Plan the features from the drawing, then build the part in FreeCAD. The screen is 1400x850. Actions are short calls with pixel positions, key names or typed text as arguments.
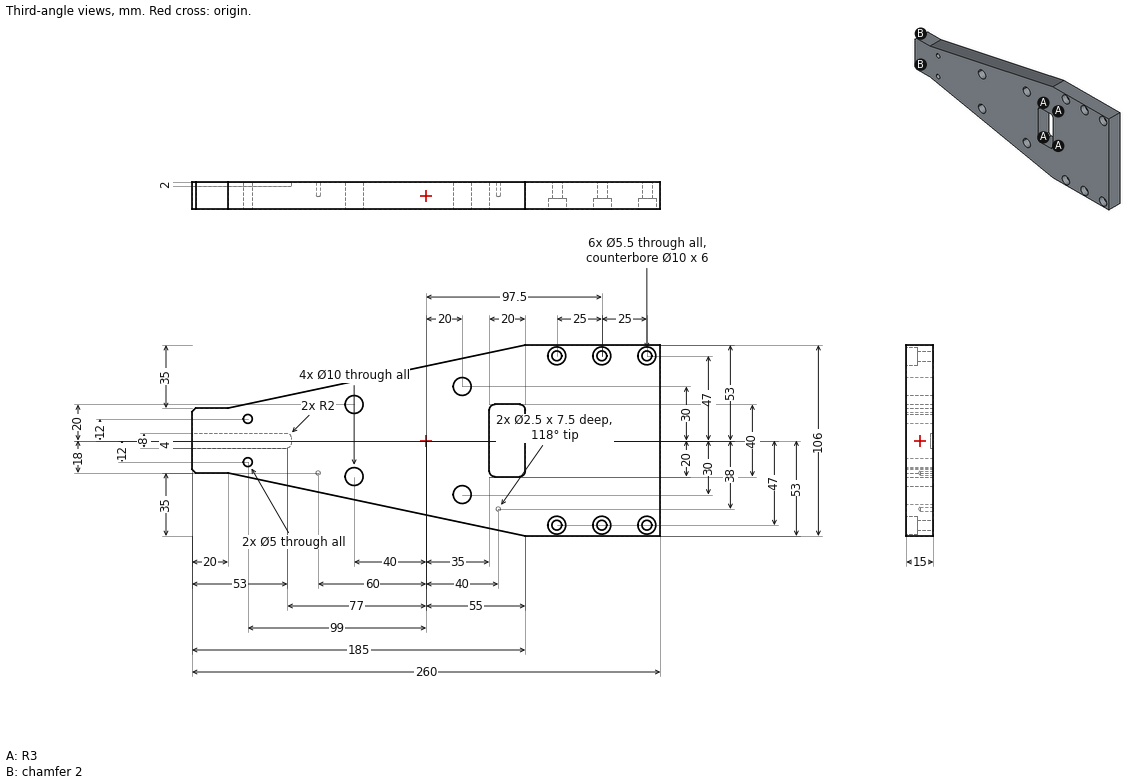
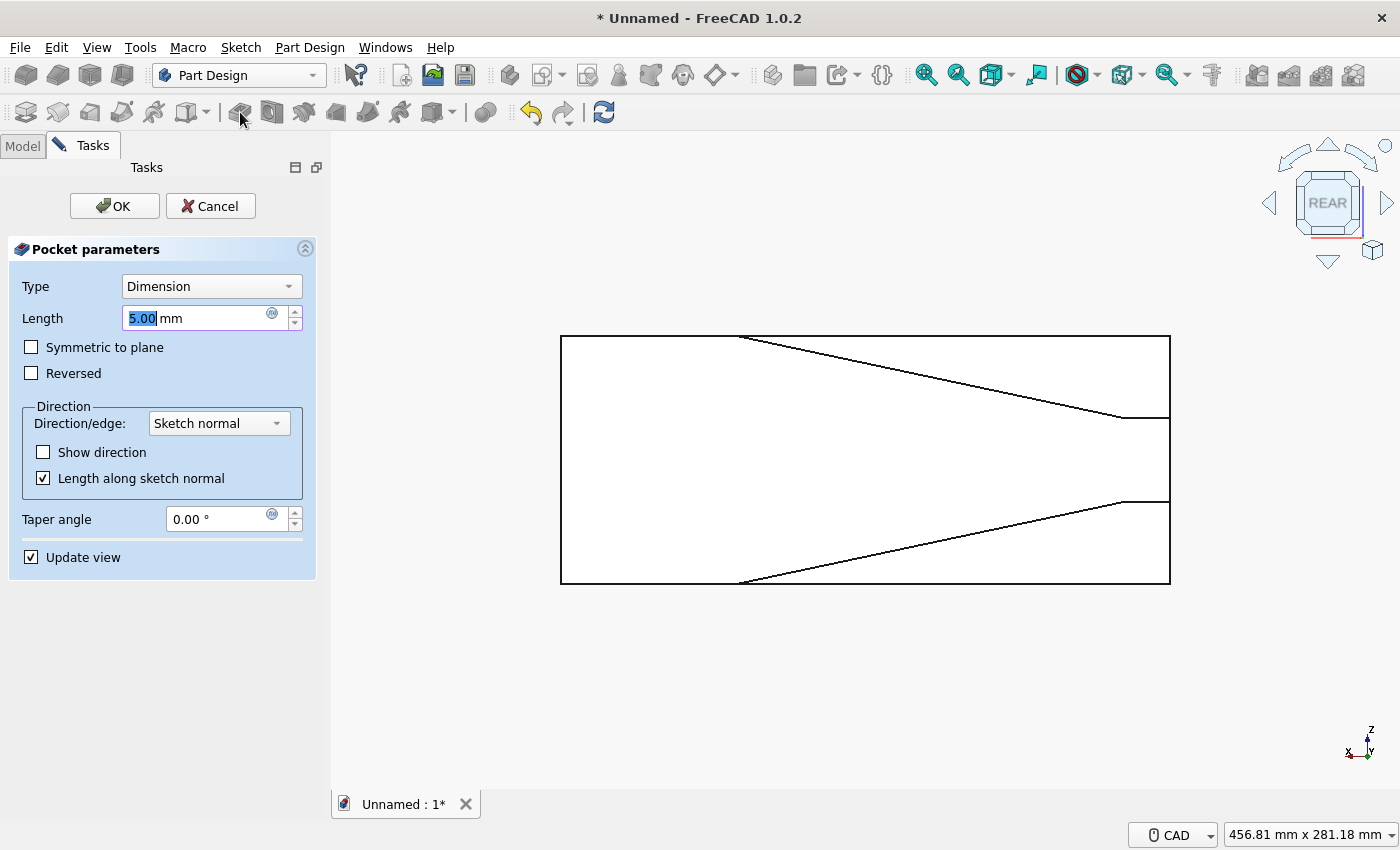
click(212, 286)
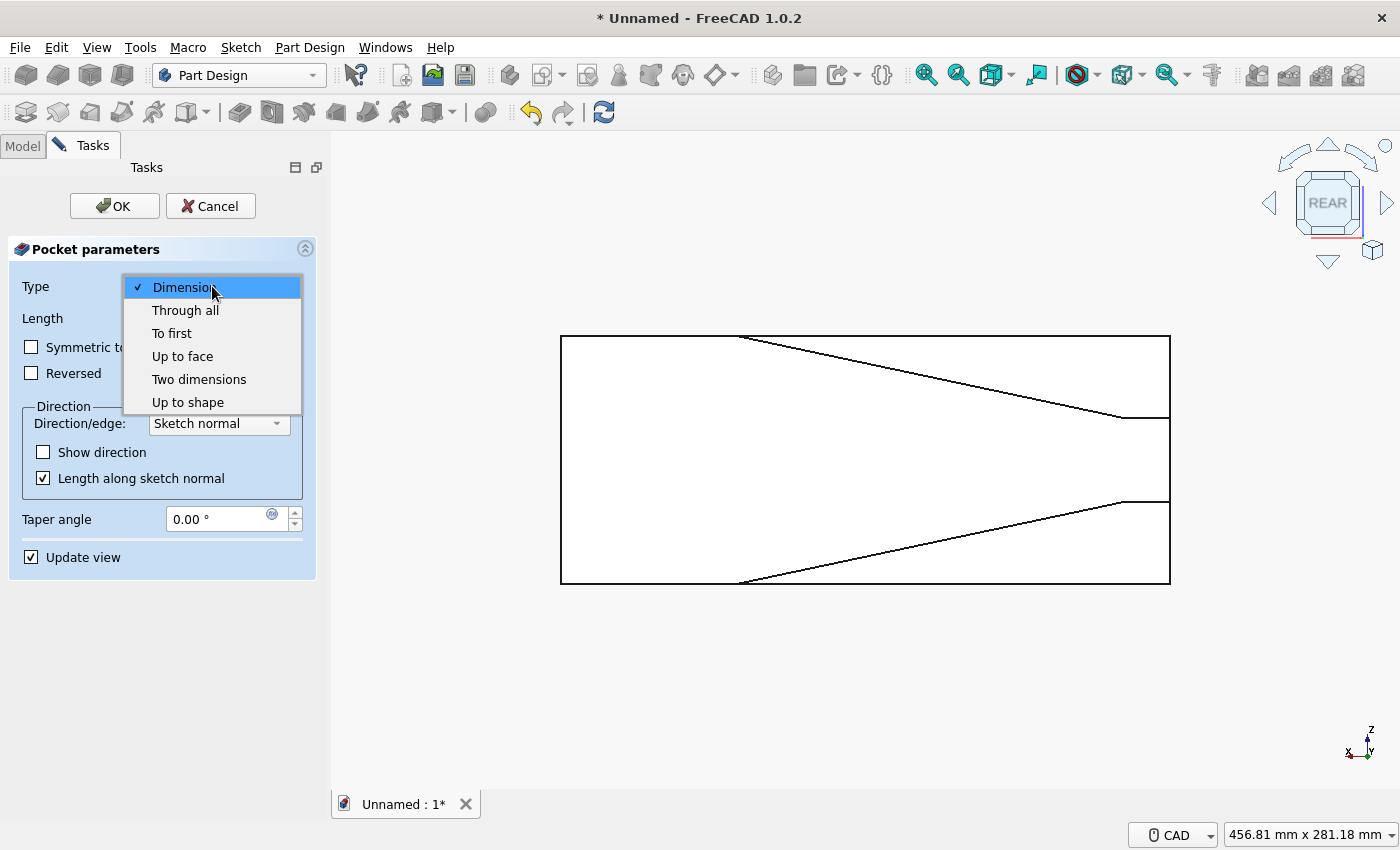
click(212, 310)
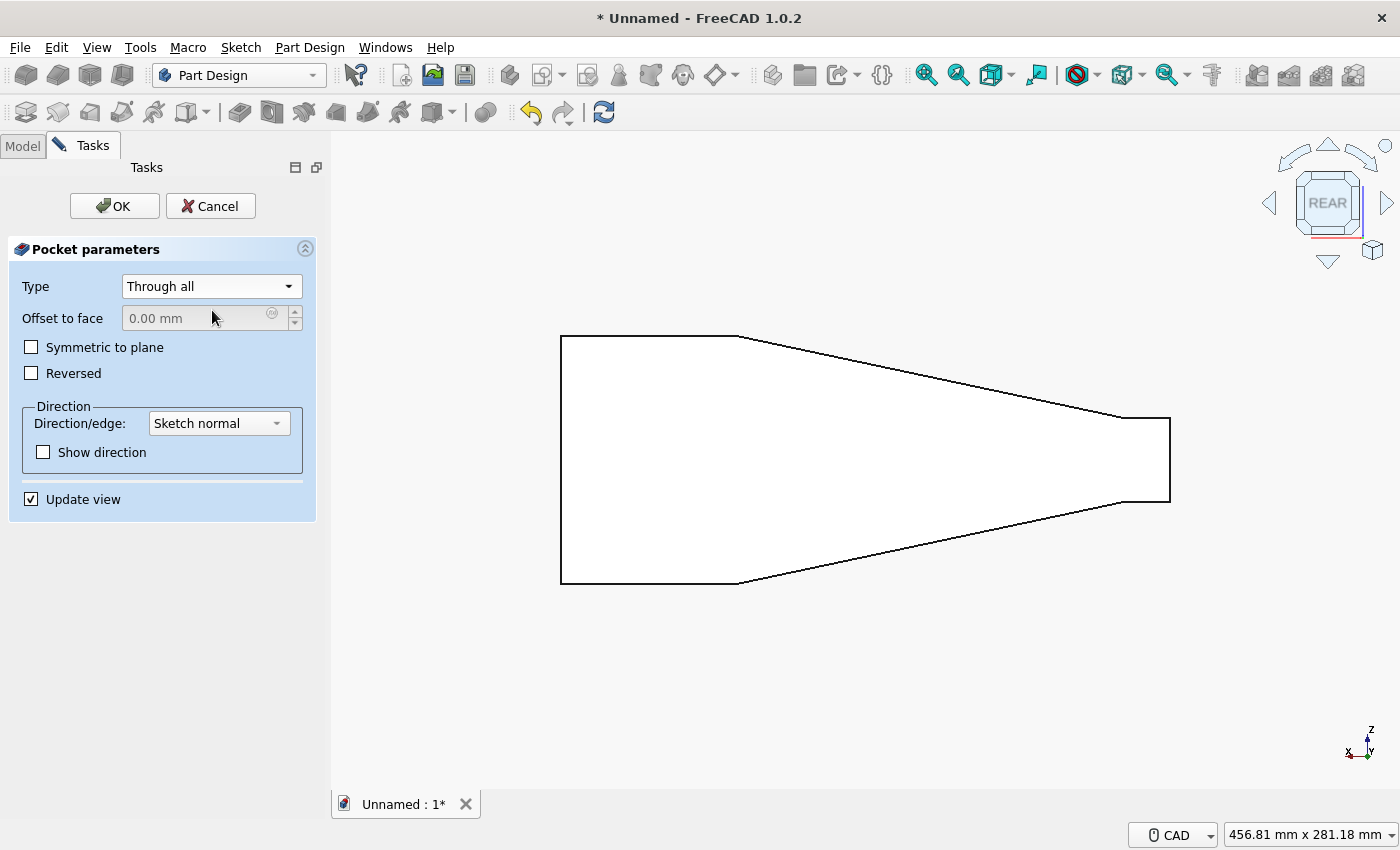
click(115, 206)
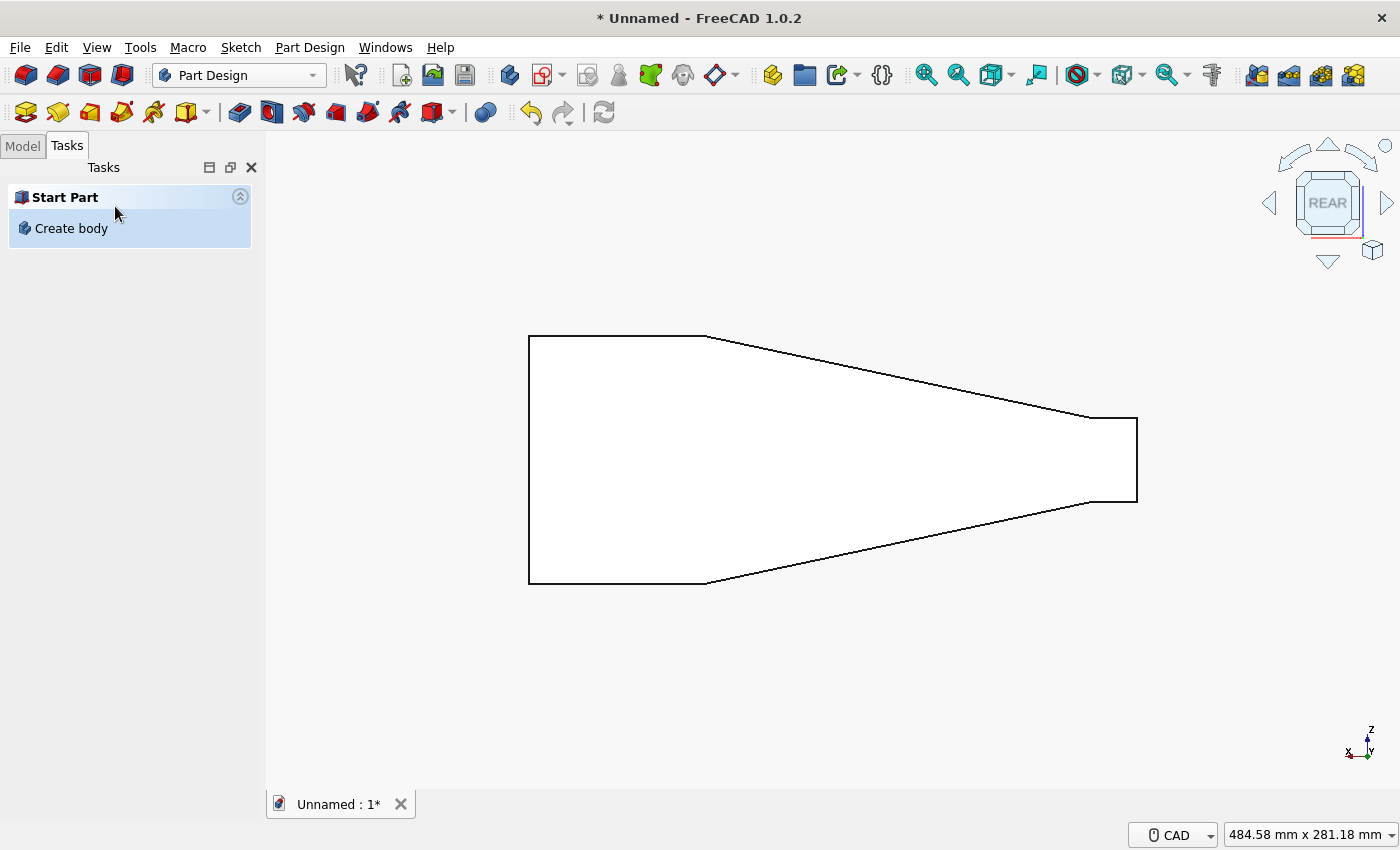
click(659, 459)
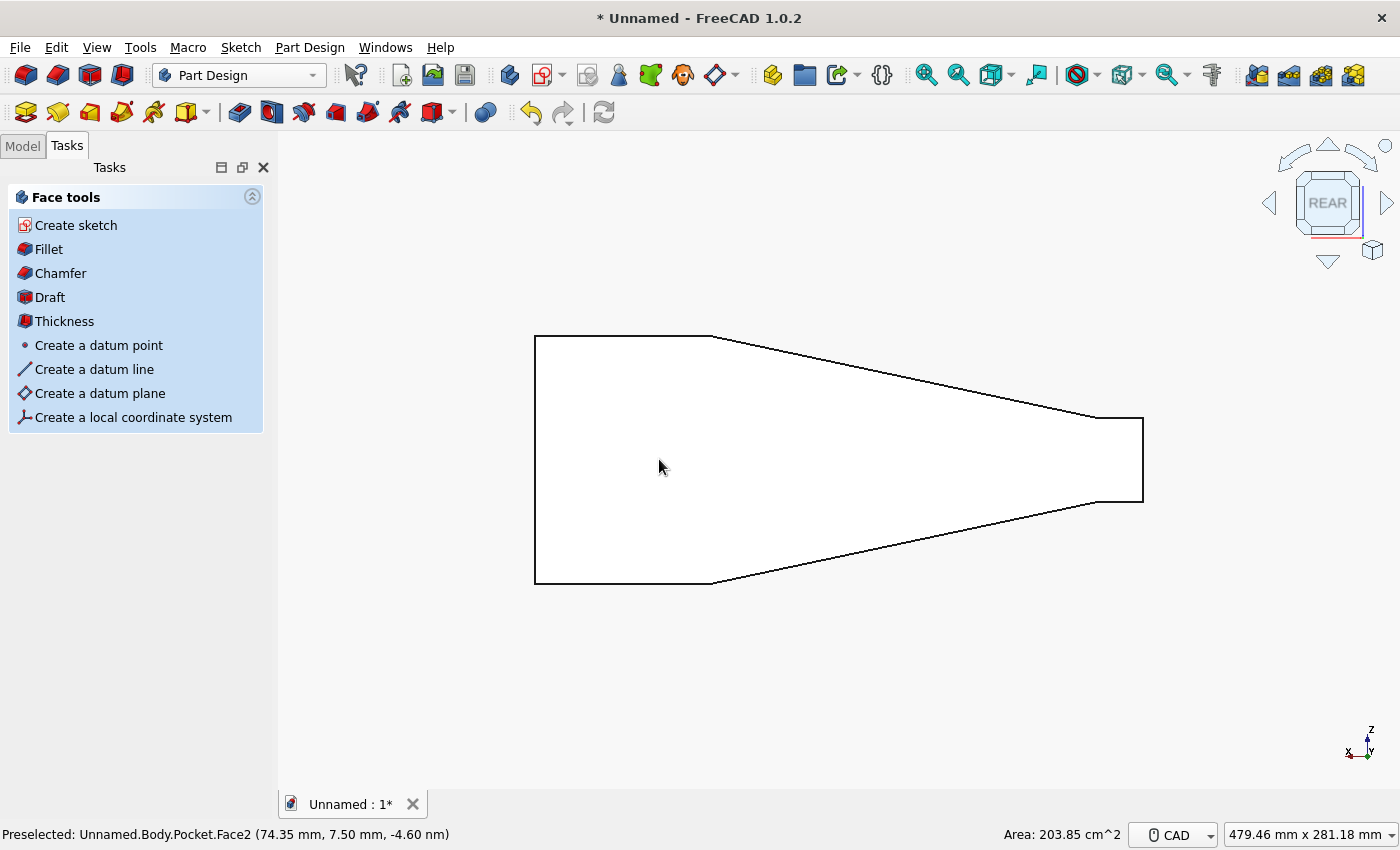
click(542, 76)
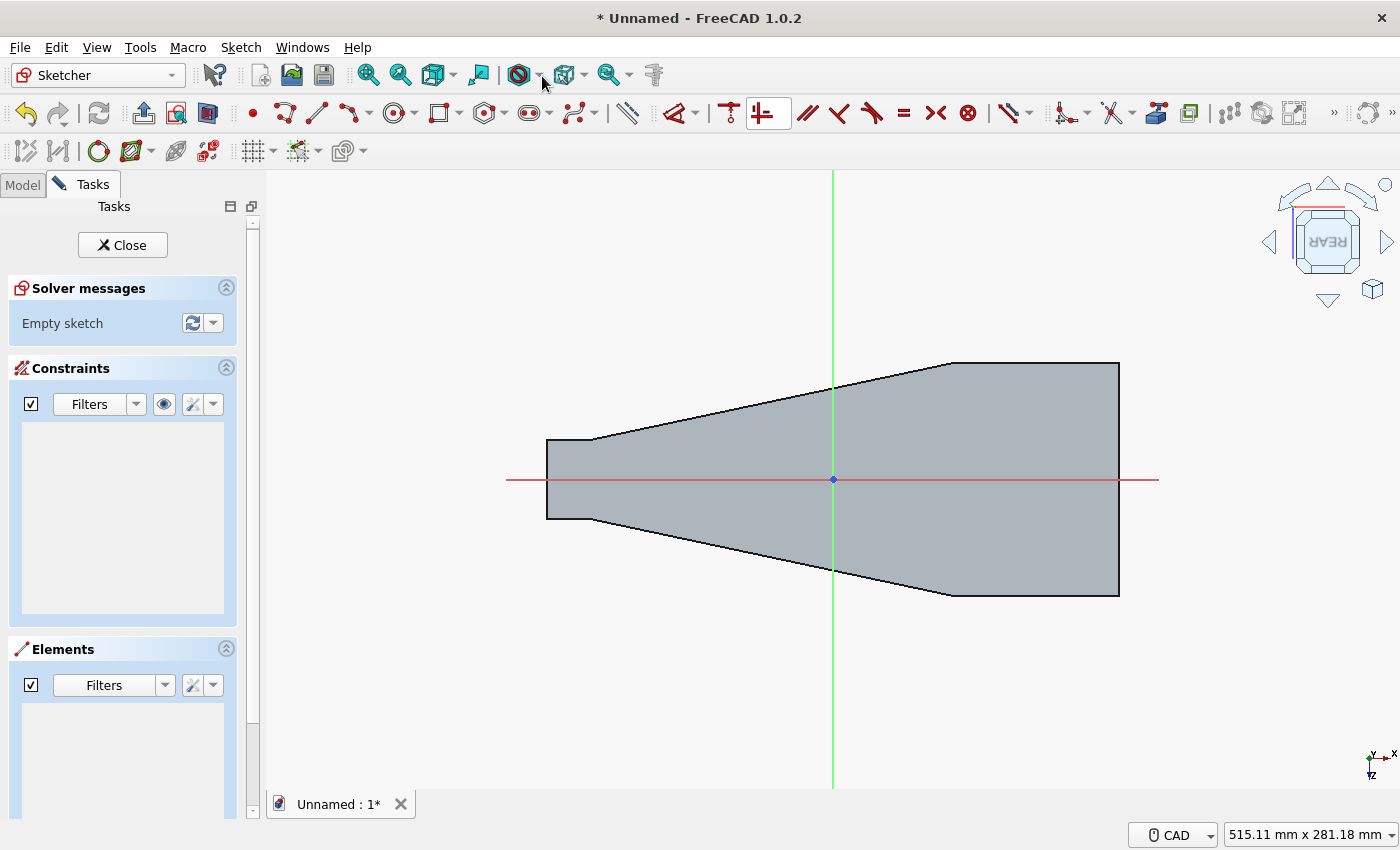
scroll(629, 479, up, 4)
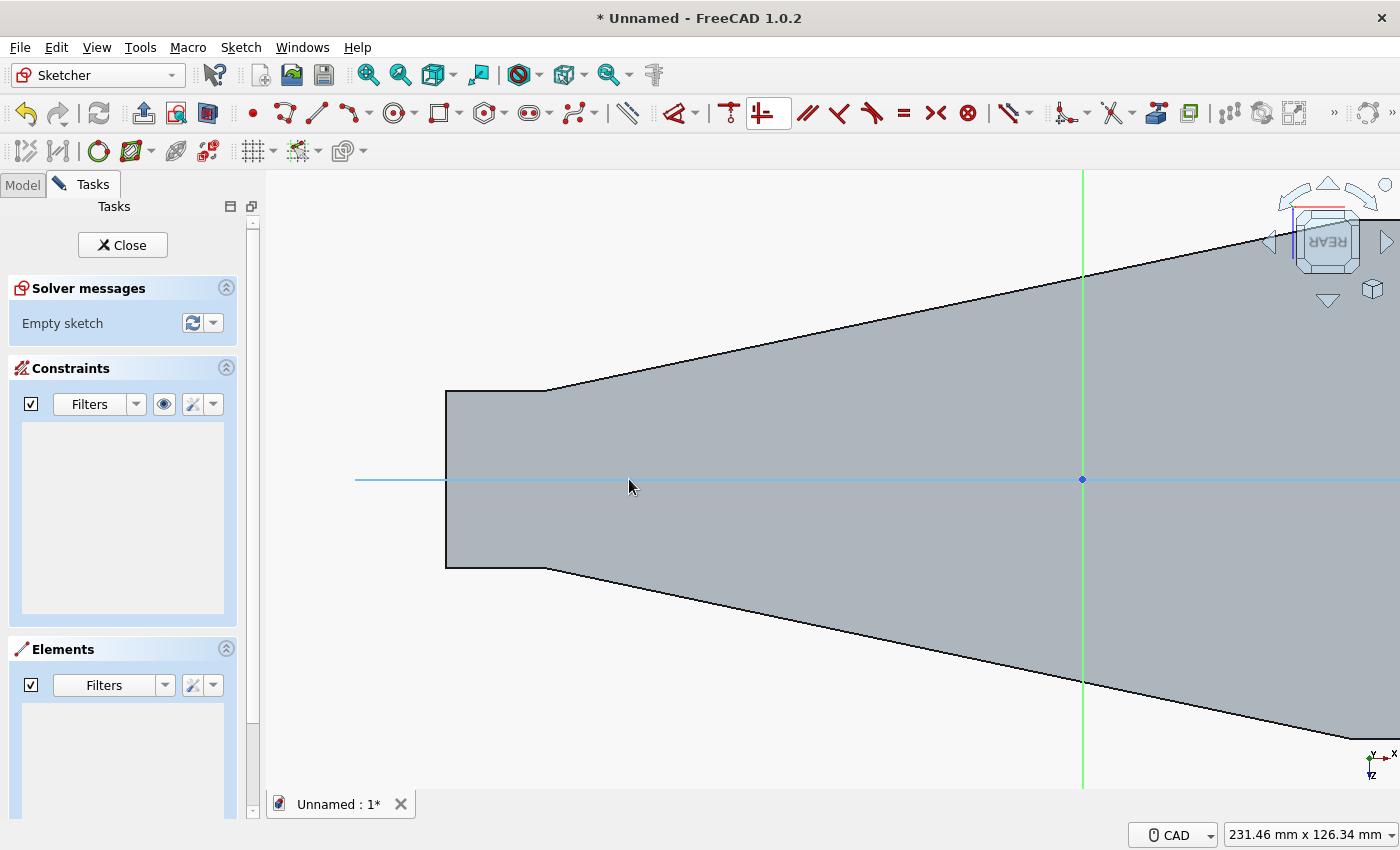
key(g)
key(m)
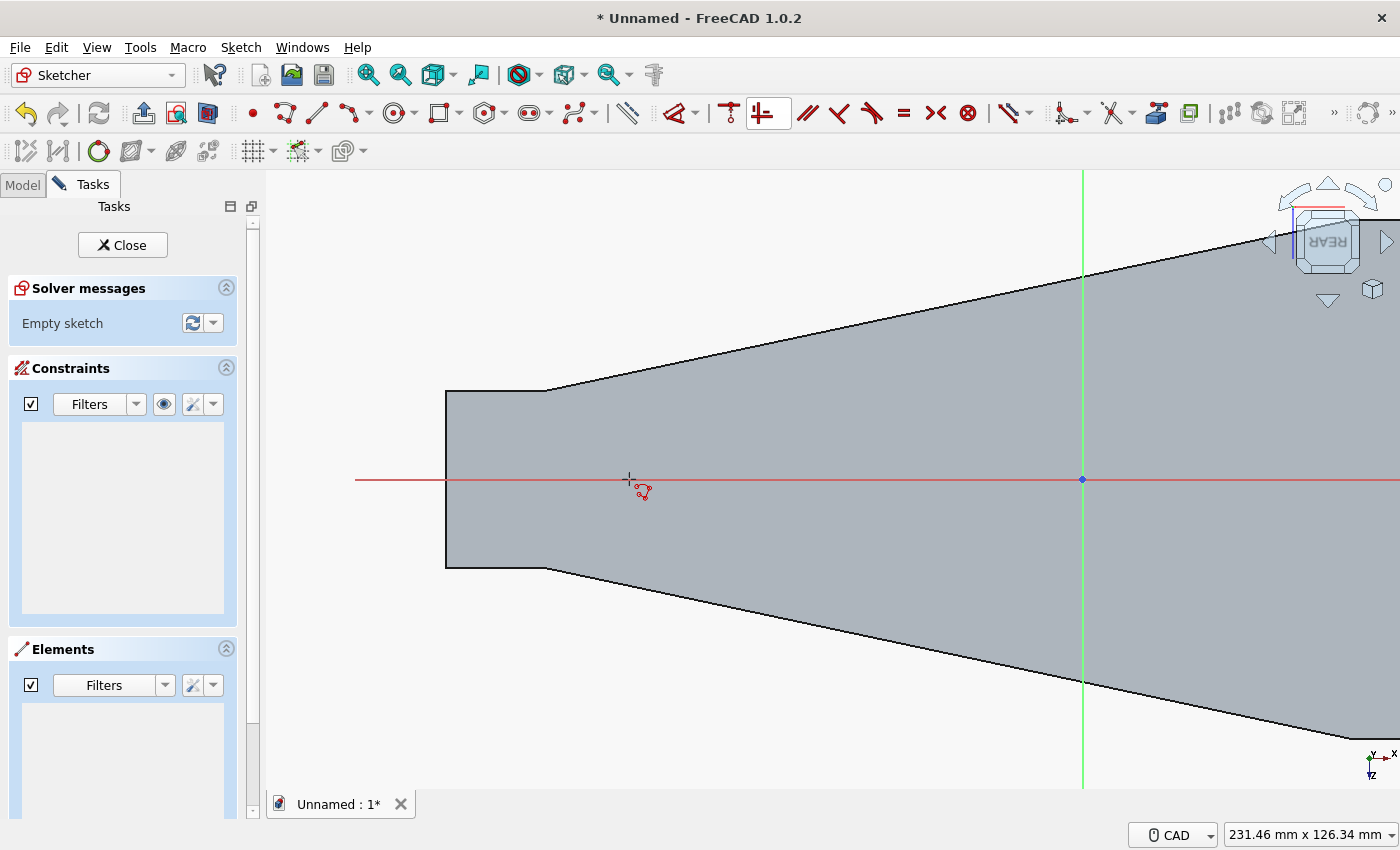
click(705, 460)
click(446, 460)
click(446, 499)
click(705, 499)
right_click(705, 499)